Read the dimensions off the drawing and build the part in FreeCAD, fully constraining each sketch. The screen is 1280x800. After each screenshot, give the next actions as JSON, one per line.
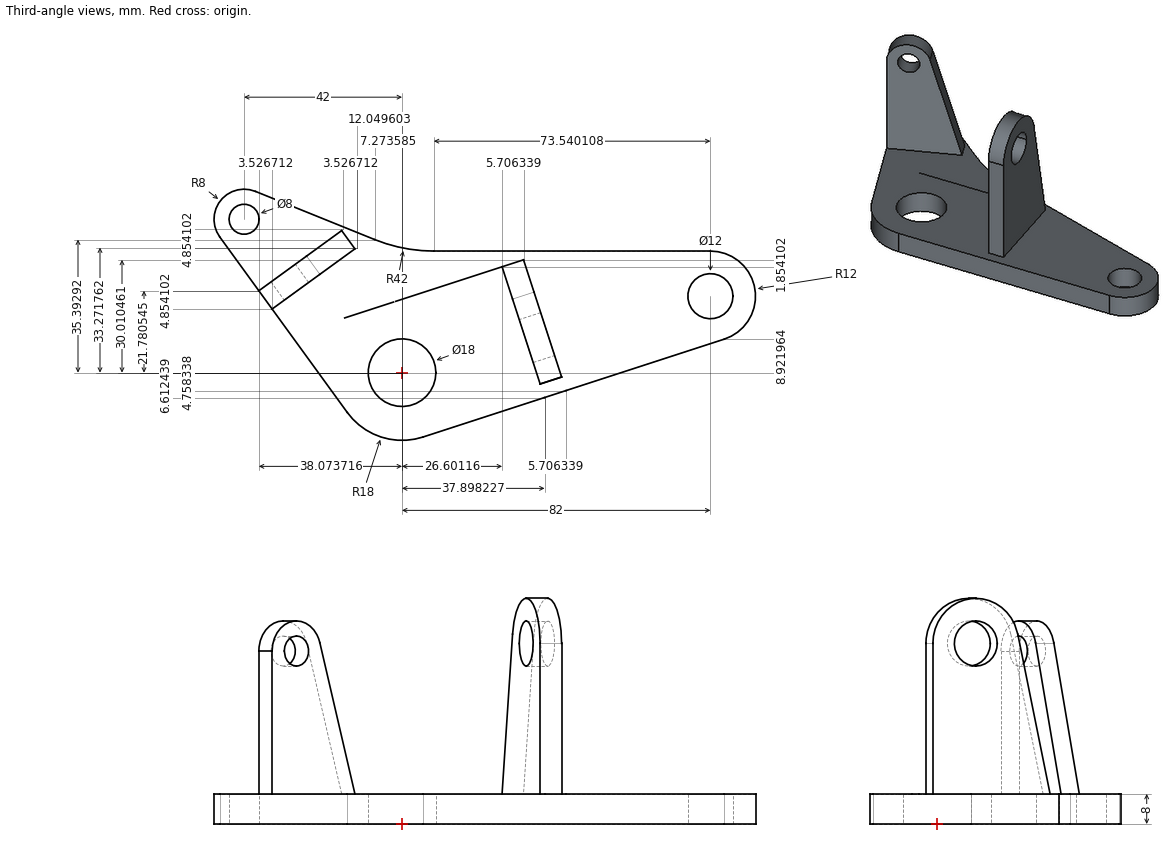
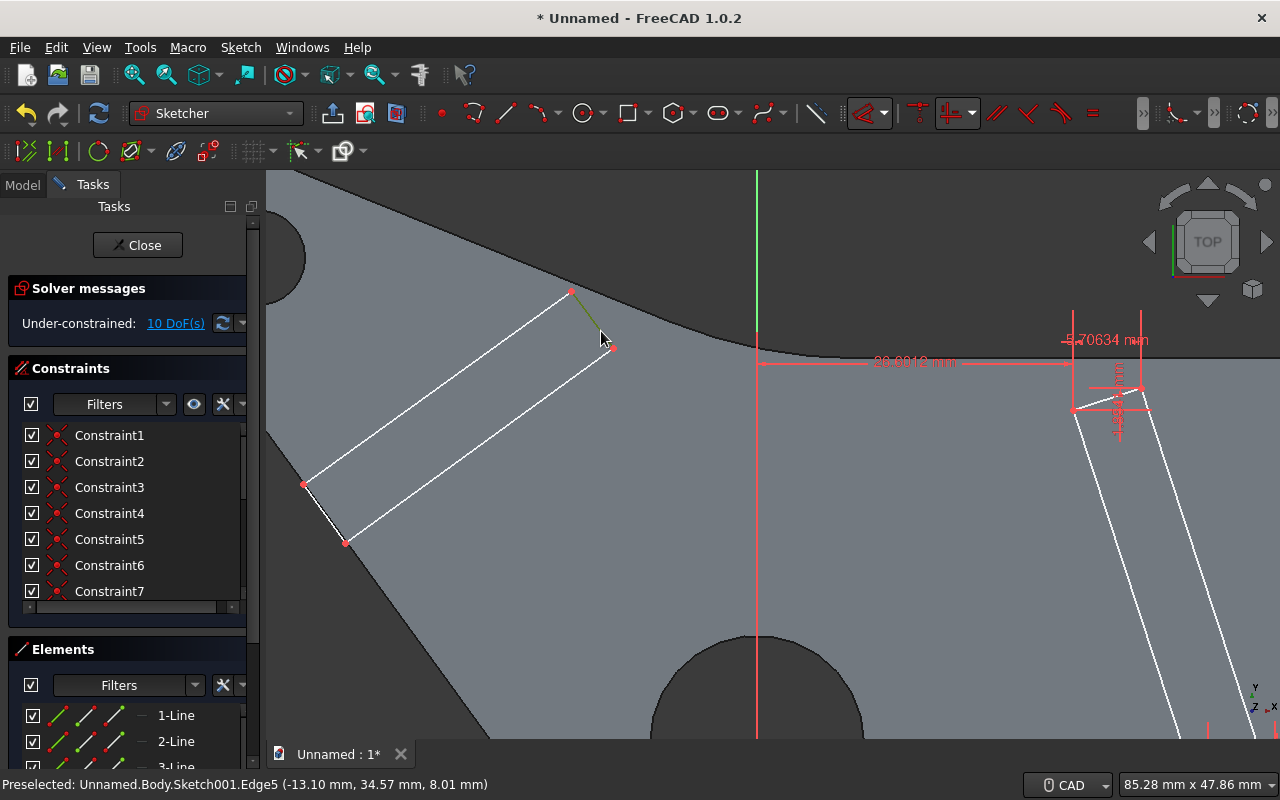
{"action": "key", "text": "l"}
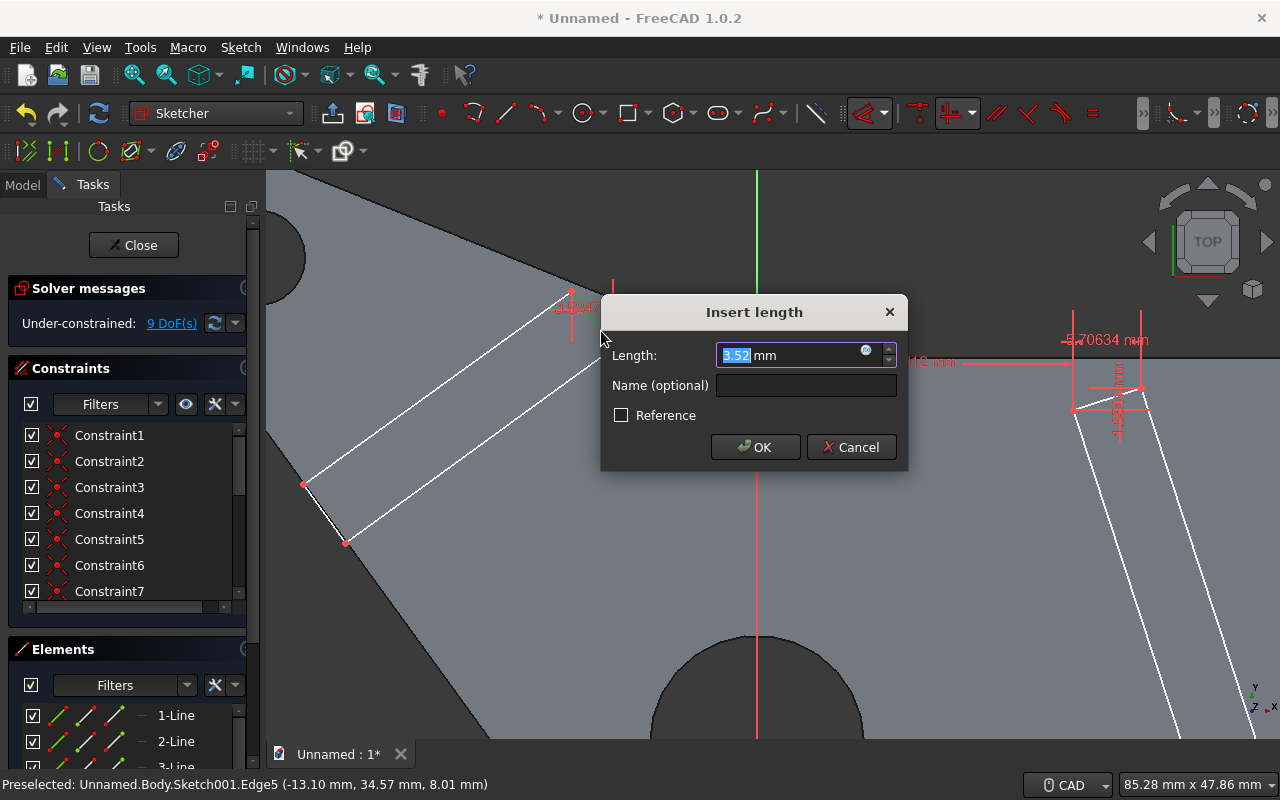
{"action": "type", "text": "3.526712"}
{"action": "key", "text": "Return"}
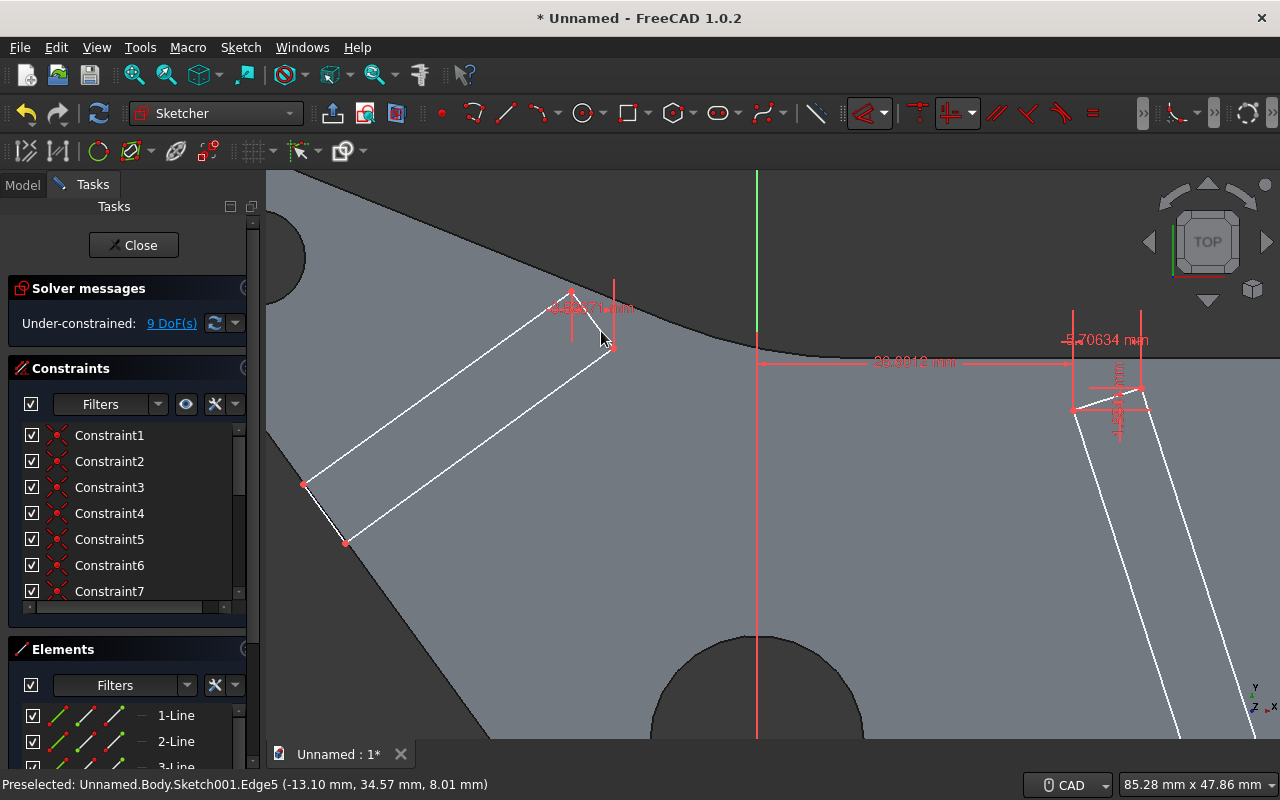
{"action": "left_click", "coordinate": [601, 331]}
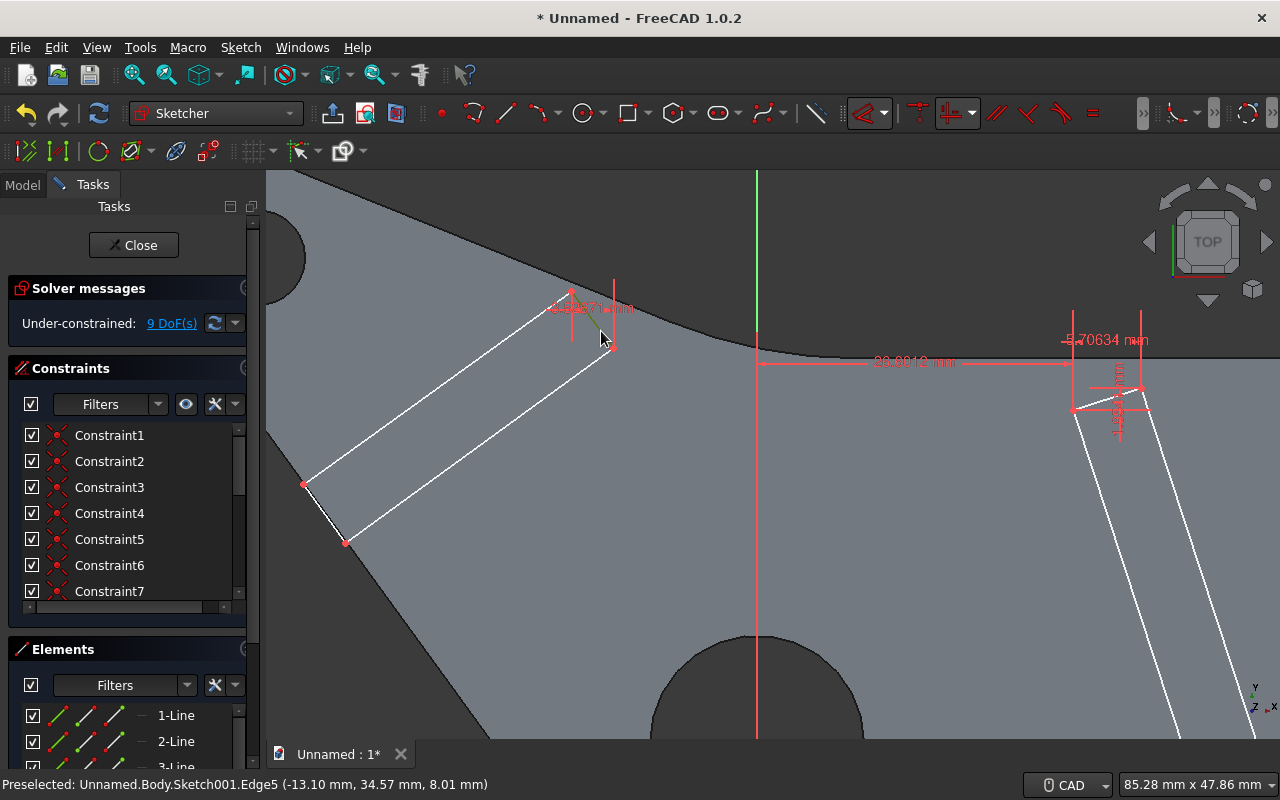
{"action": "key", "text": "i"}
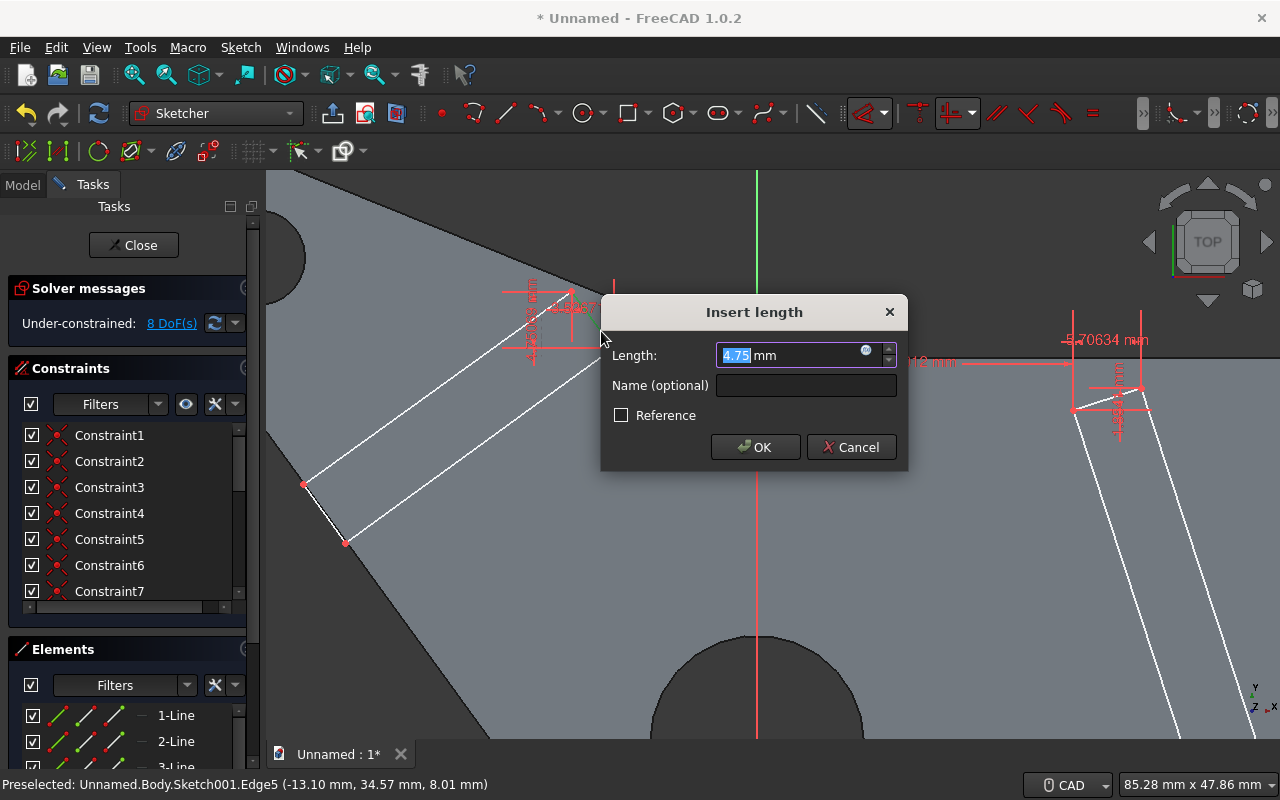
{"action": "type", "text": "4.854102"}
{"action": "key", "text": "Return"}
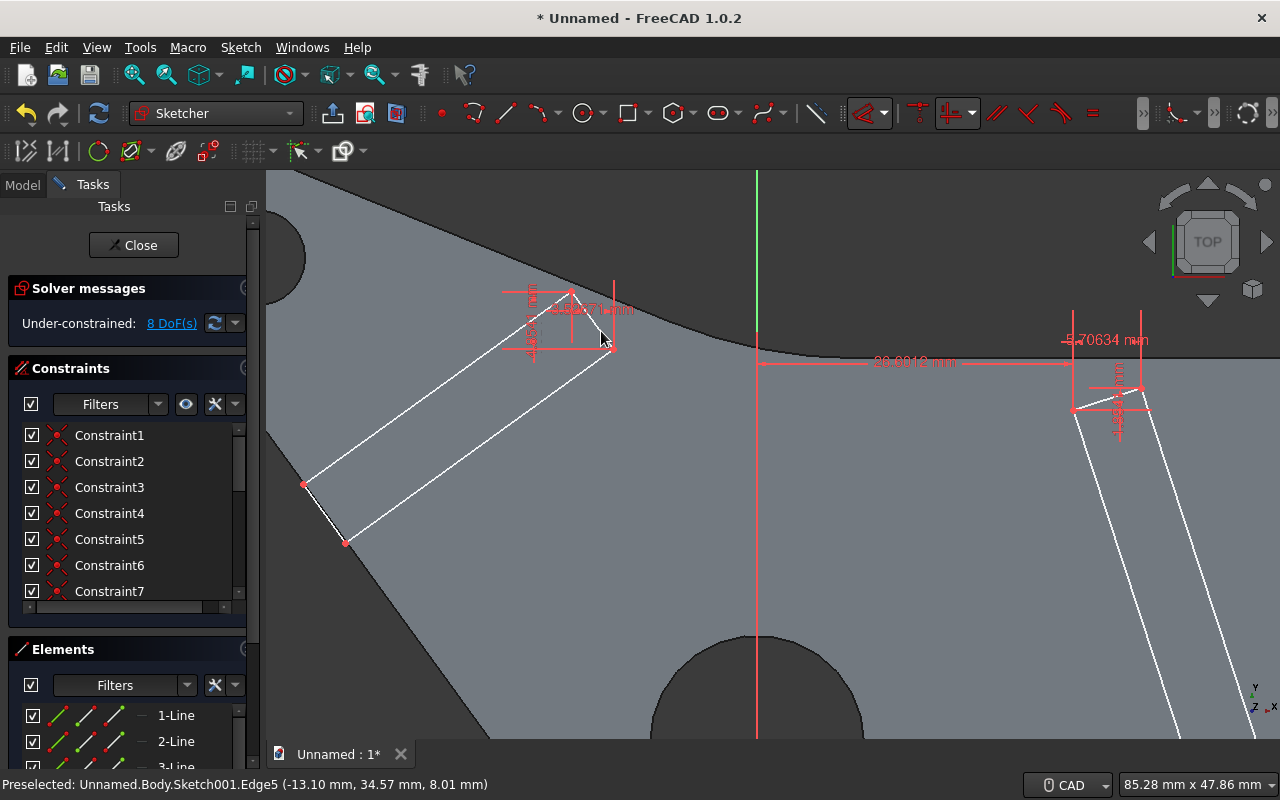
{"action": "left_click", "coordinate": [316, 502]}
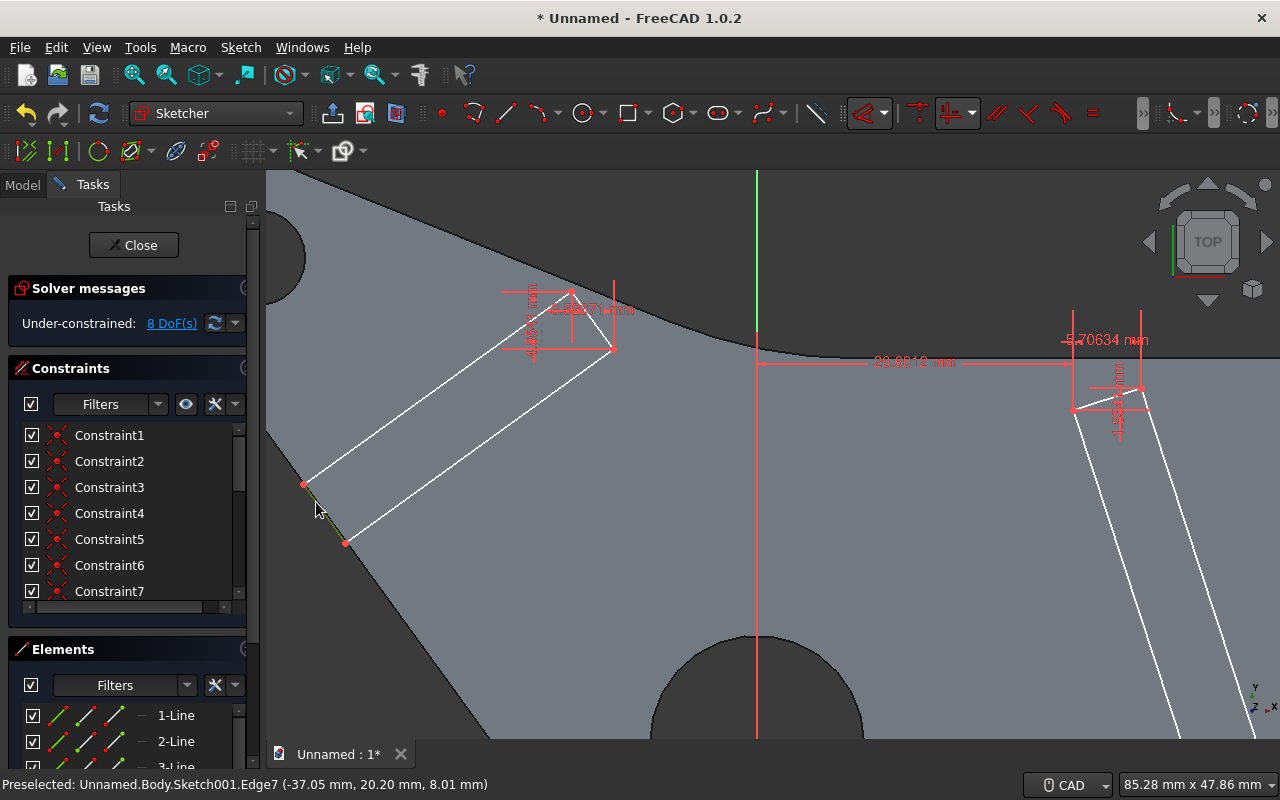
{"action": "key", "text": "l"}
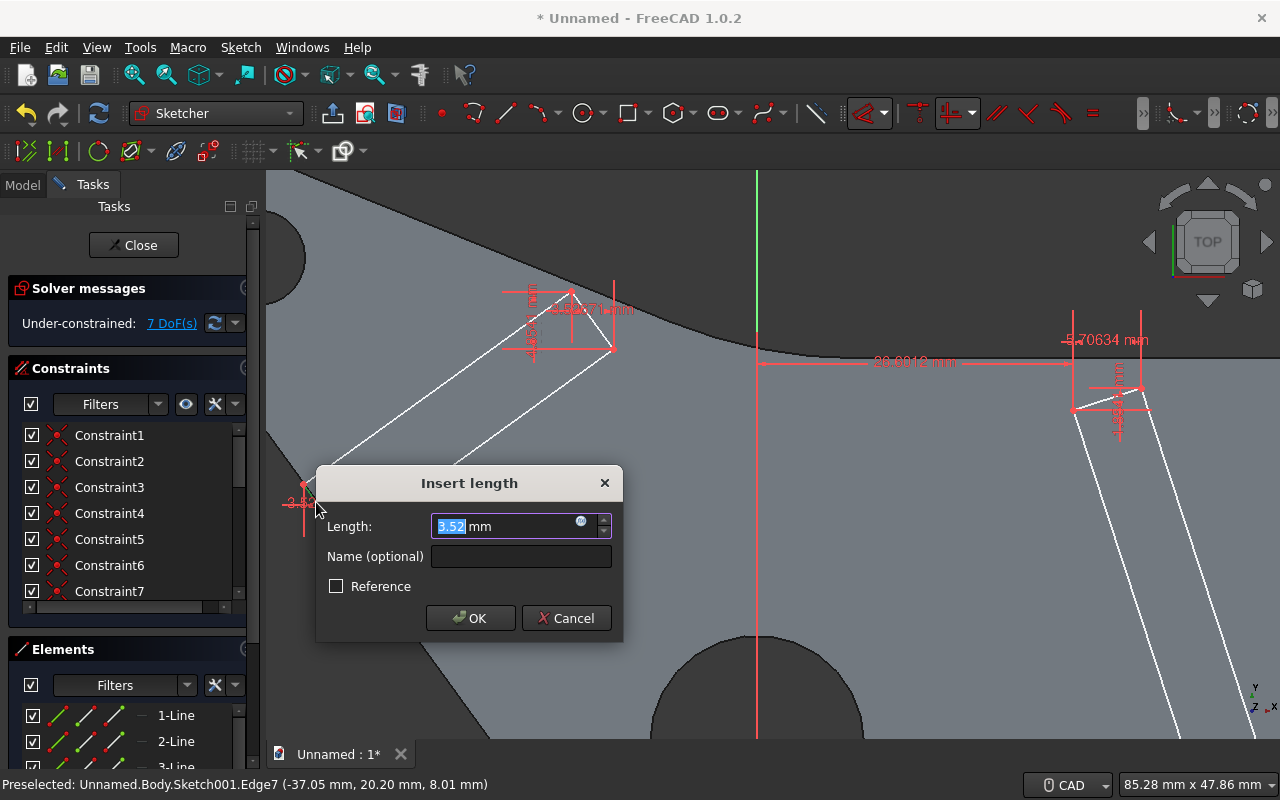
{"action": "type", "text": "3.526712"}
{"action": "key", "text": "Return"}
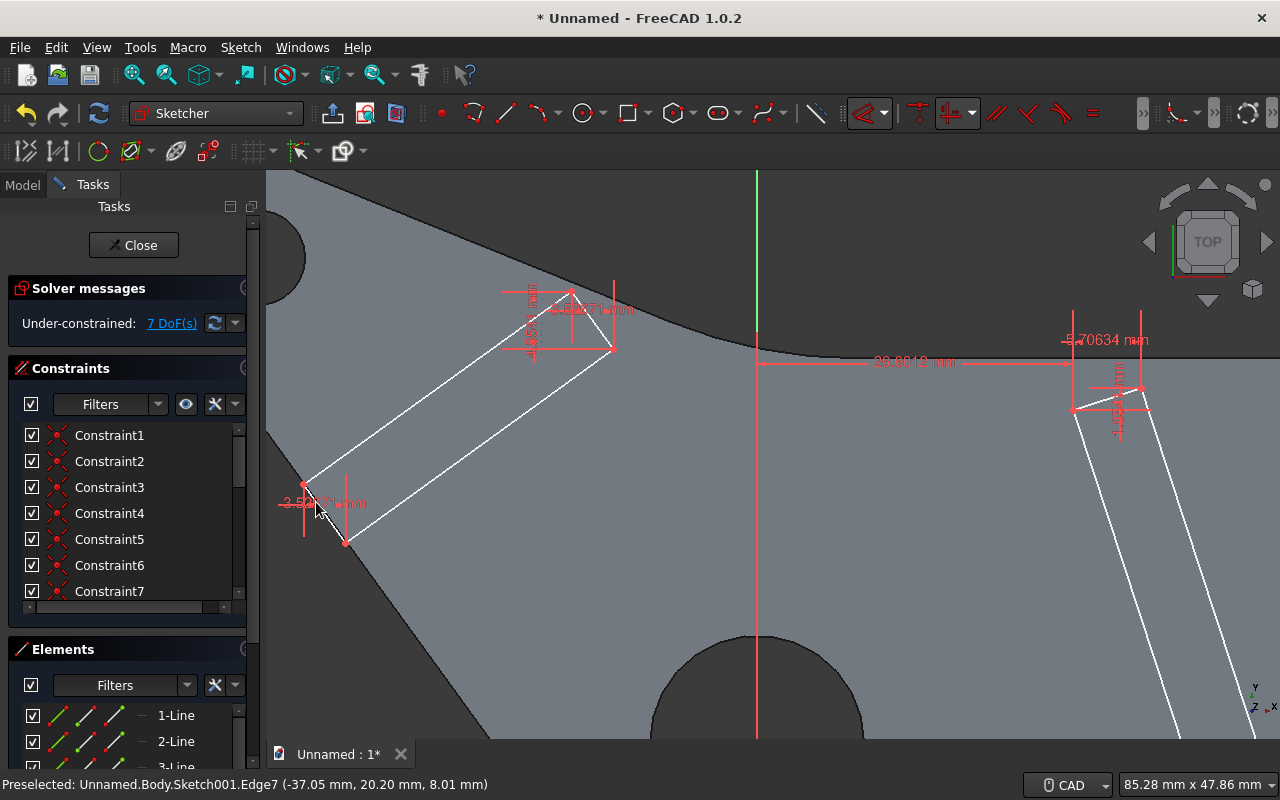
{"action": "left_click", "coordinate": [333, 526]}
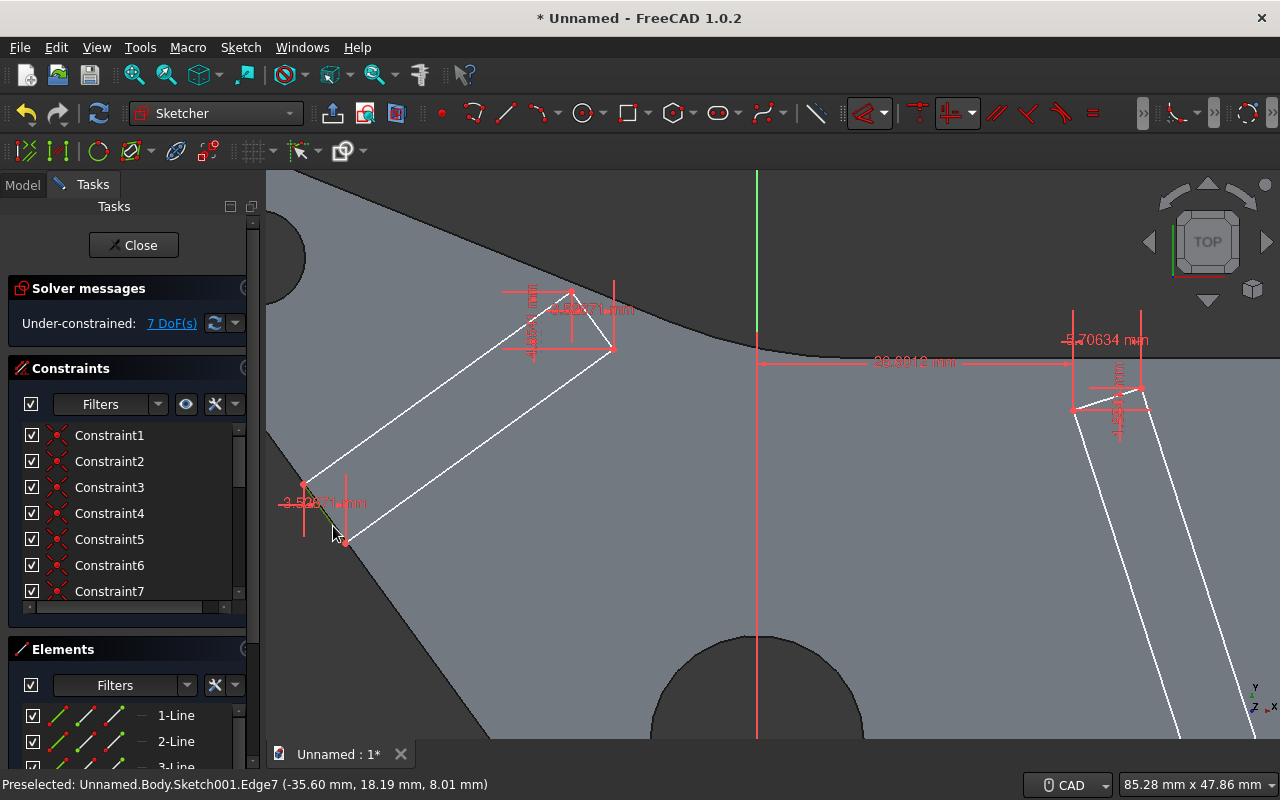
{"action": "left_click", "coordinate": [886, 114]}